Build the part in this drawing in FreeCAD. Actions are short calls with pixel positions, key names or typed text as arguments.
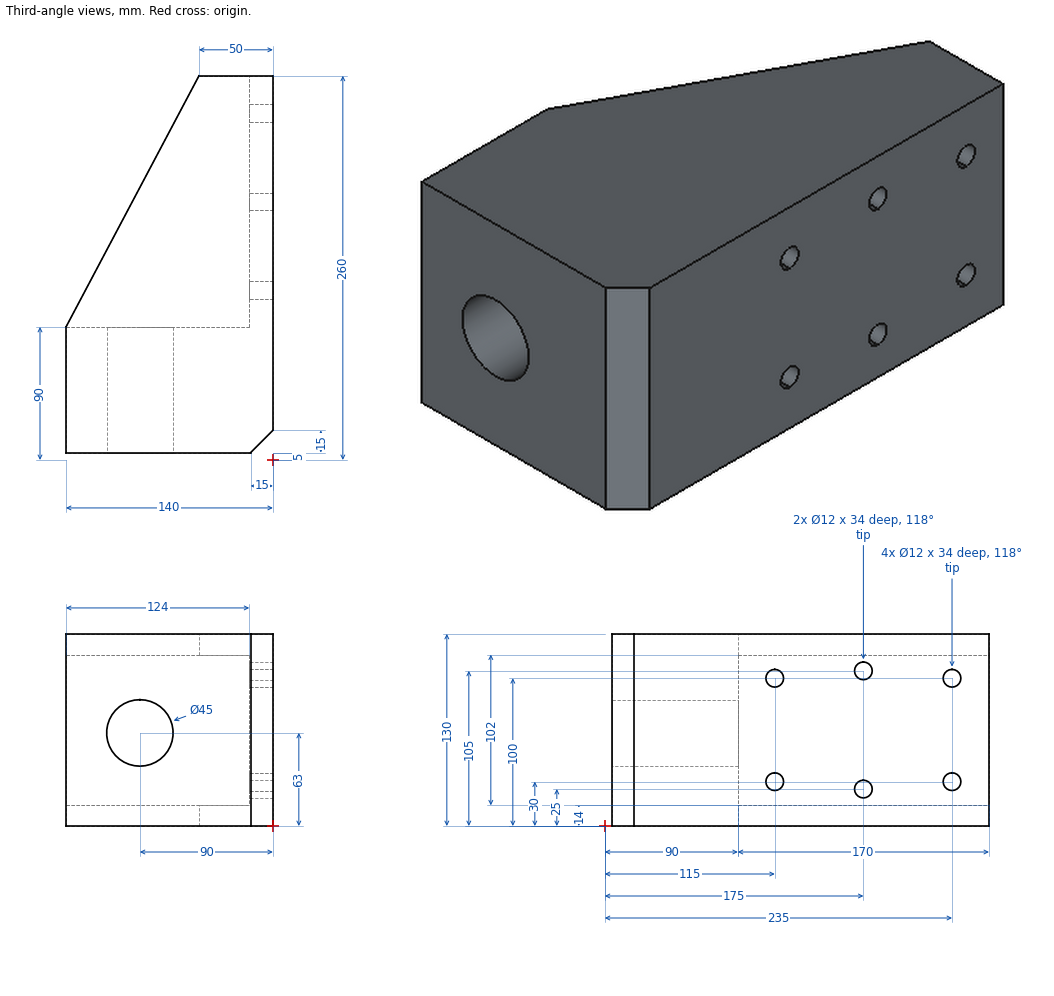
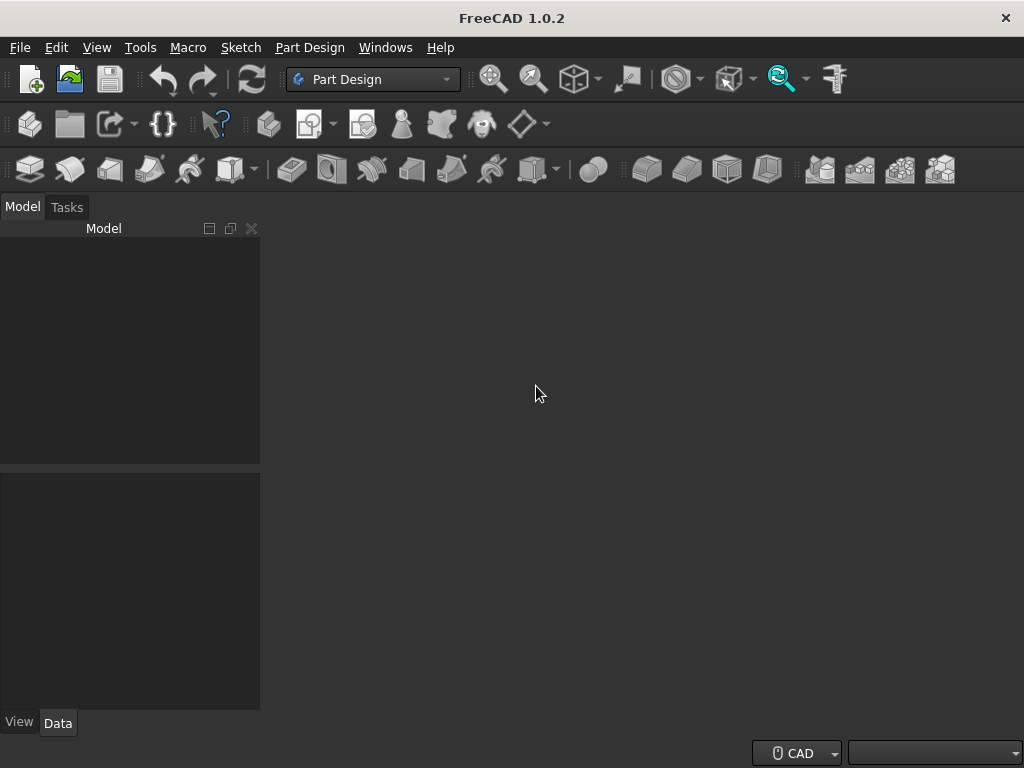
click(30, 80)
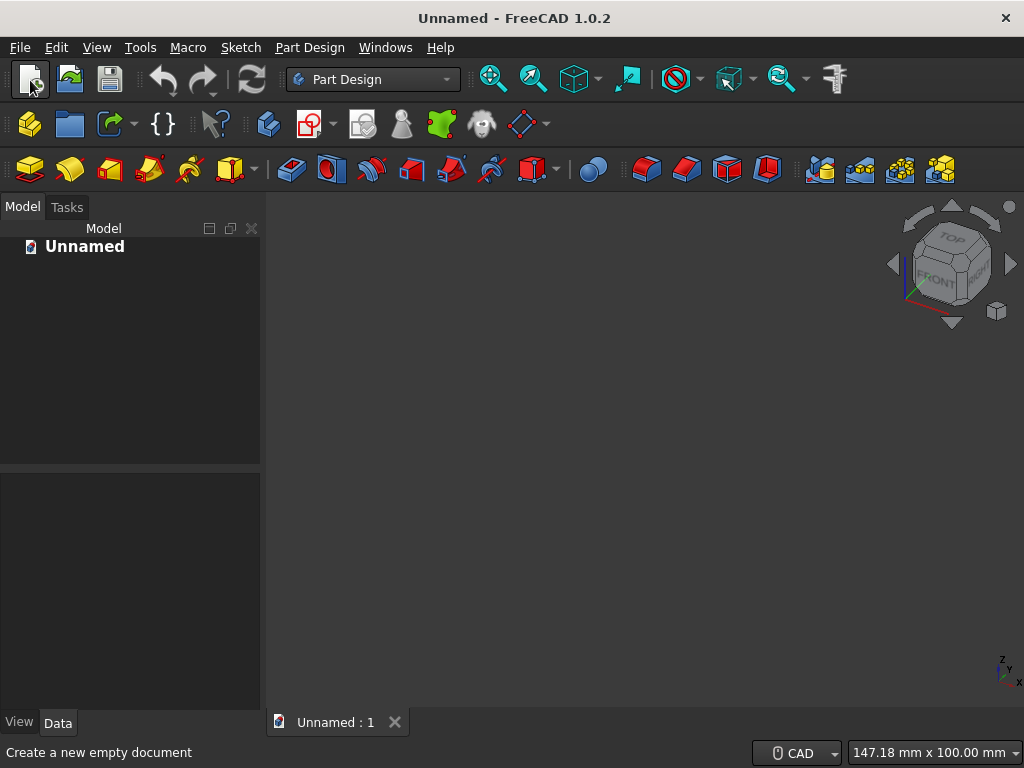
click(310, 124)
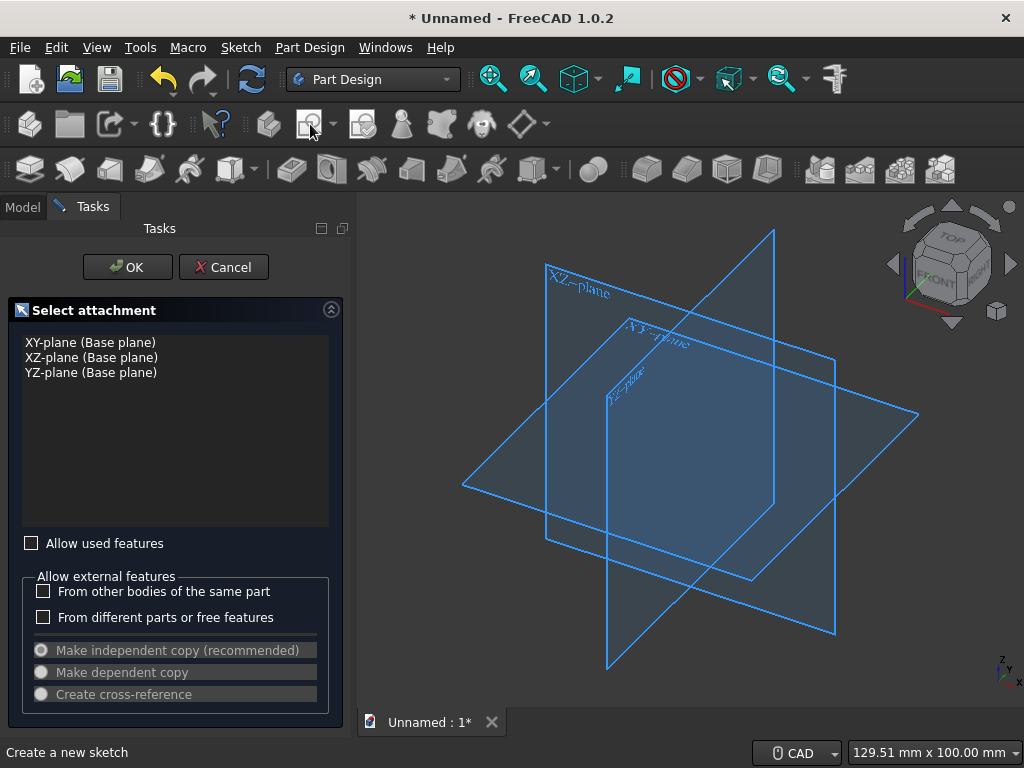
click(82, 342)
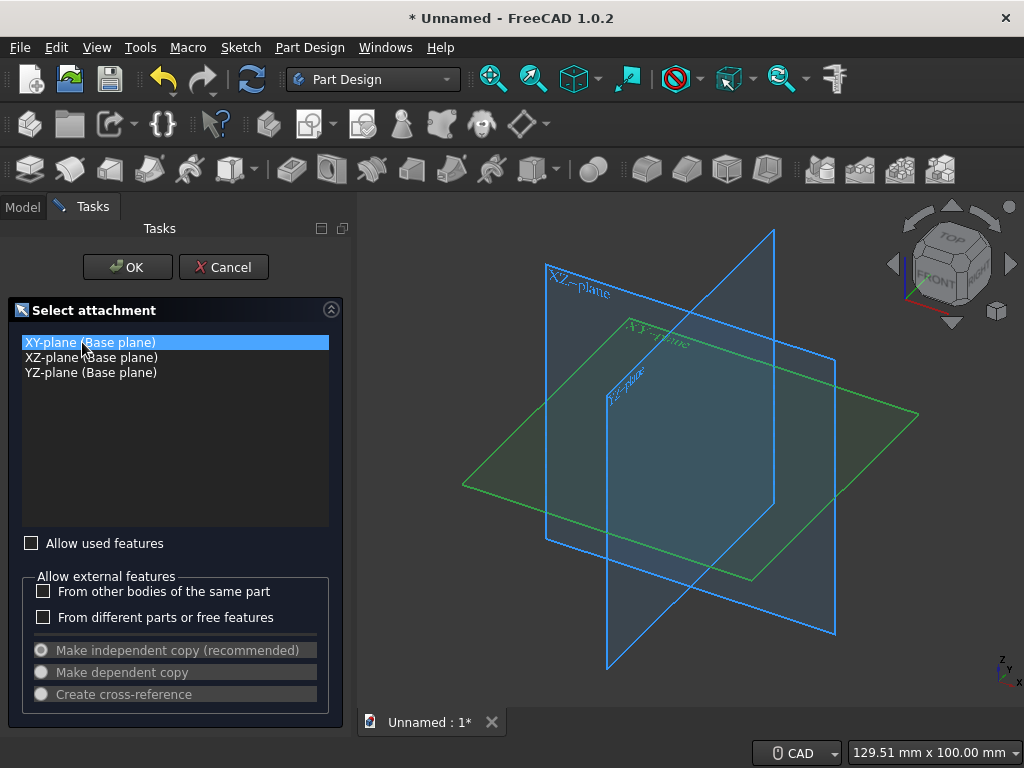
click(128, 267)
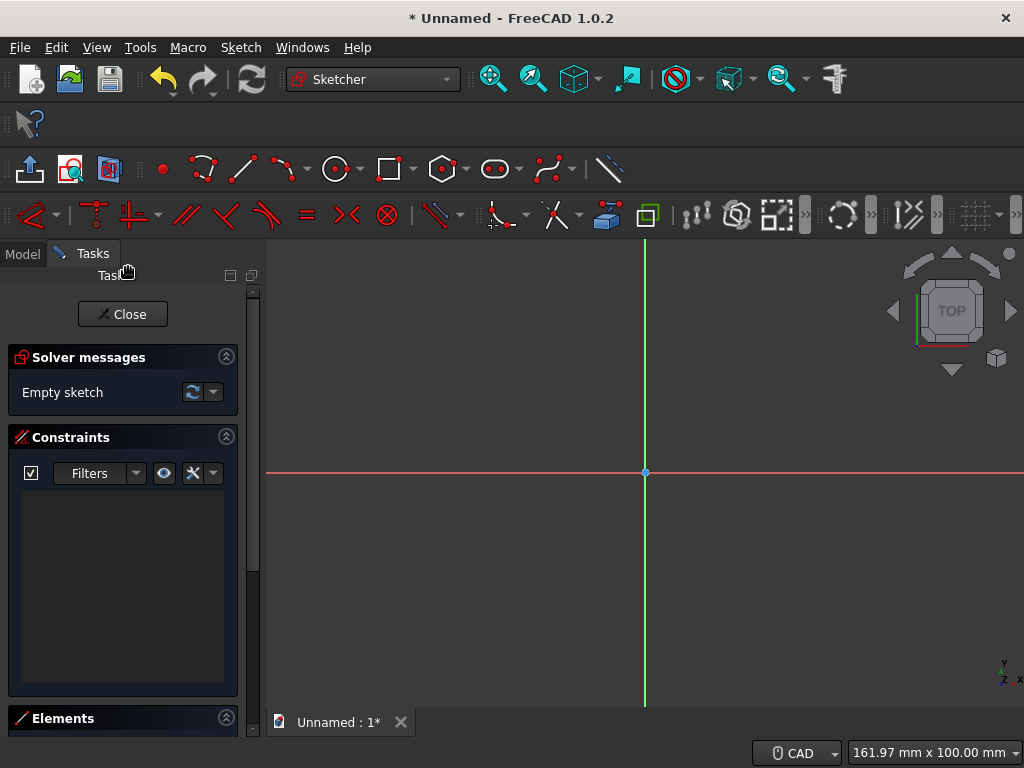
scroll(661, 672, down, 7)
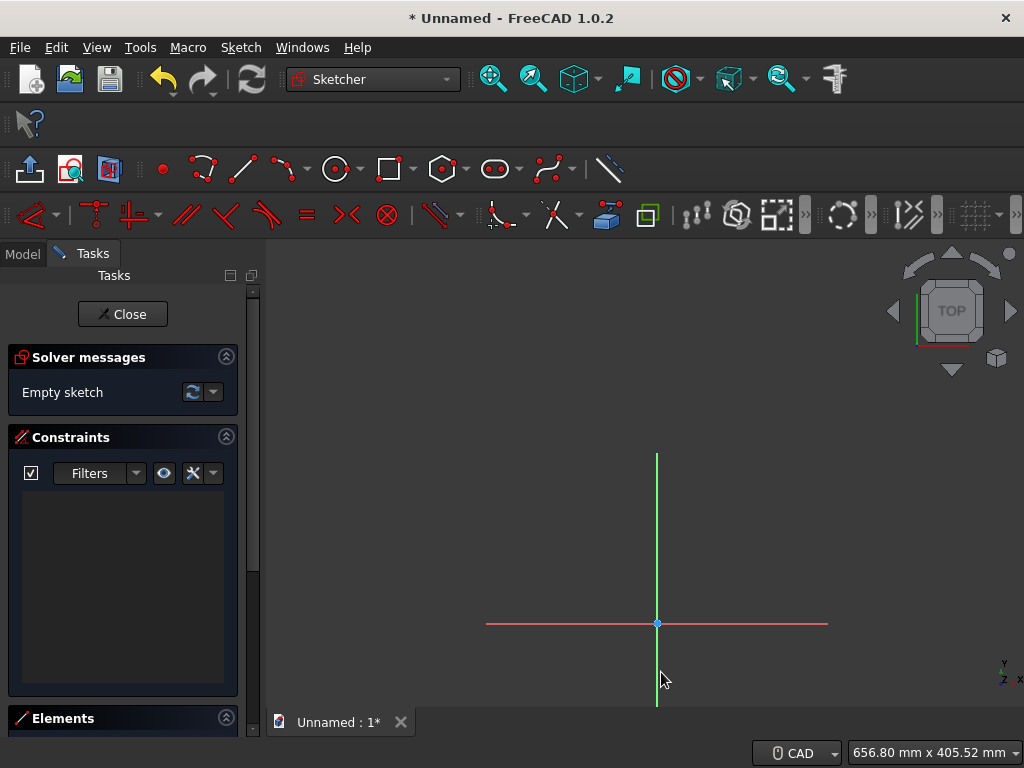
click(204, 170)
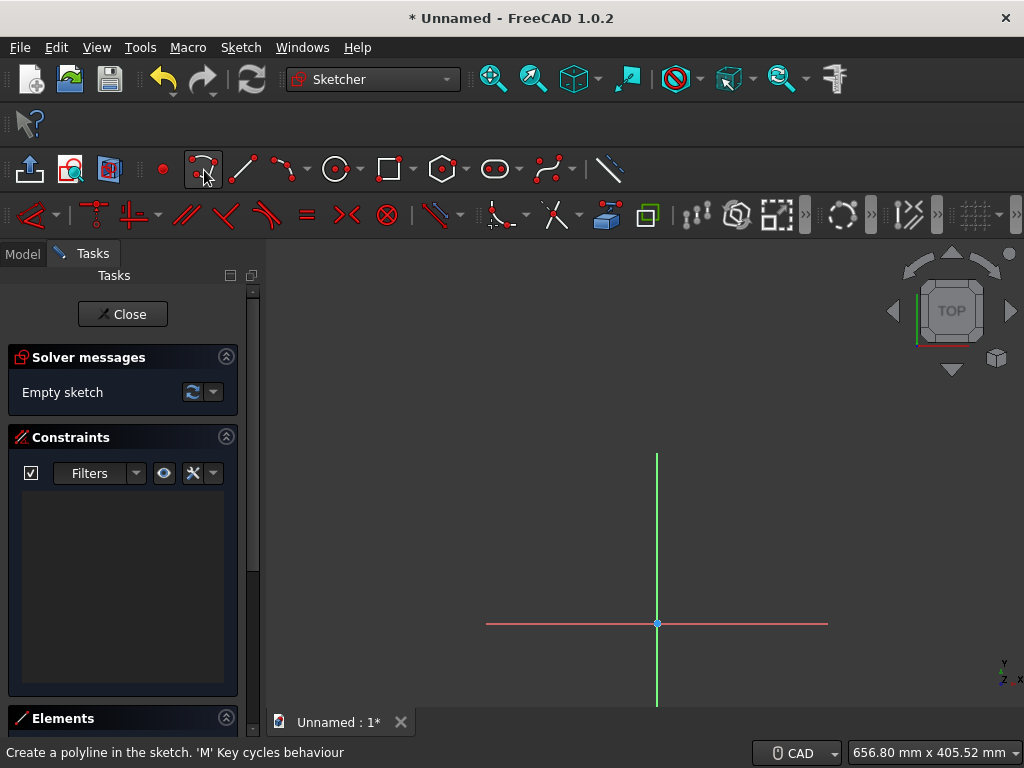
click(657, 624)
click(648, 324)
click(600, 324)
click(496, 520)
click(496, 615)
click(657, 624)
key(Escape)
key(Escape)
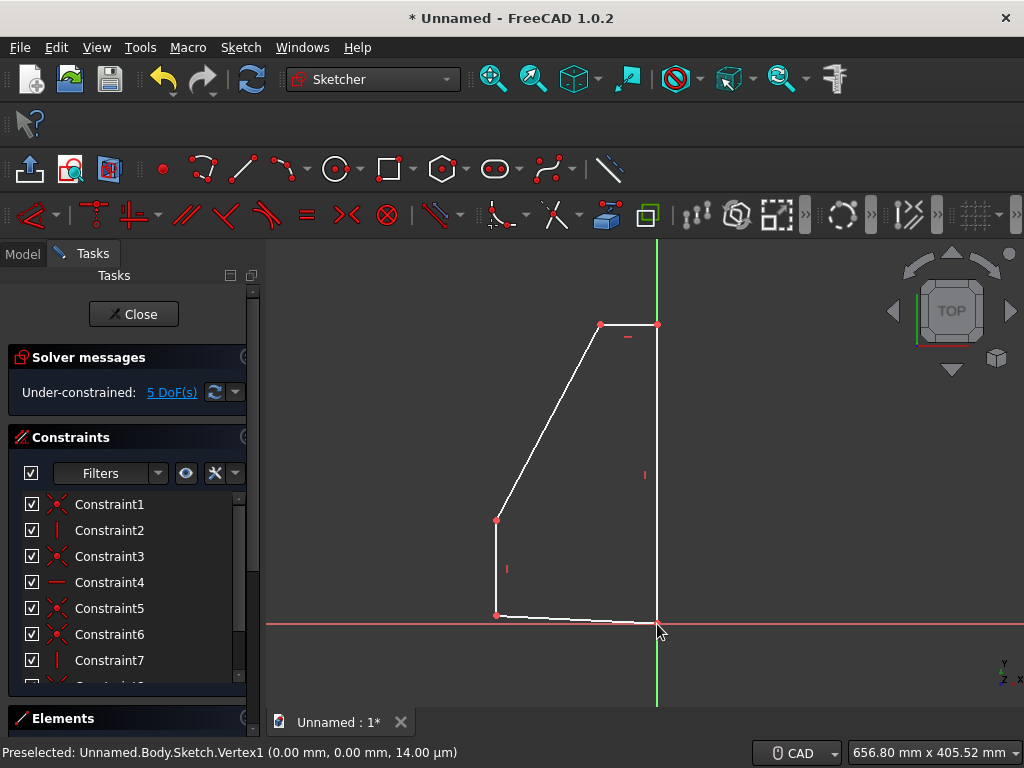
click(609, 621)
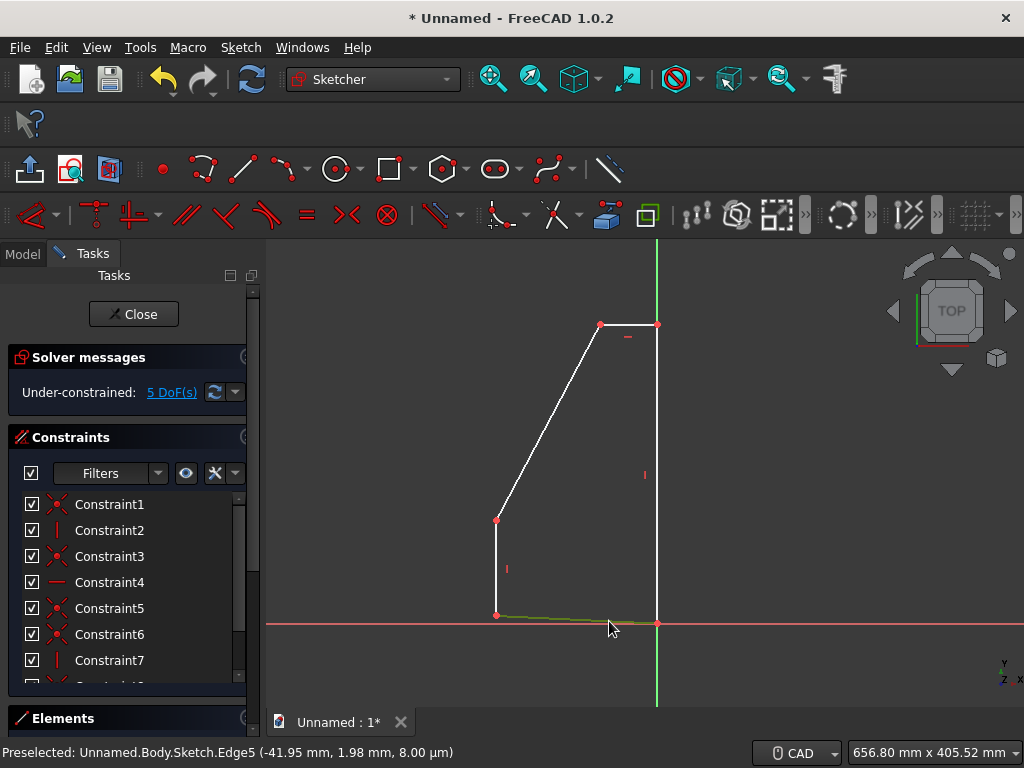
key(h)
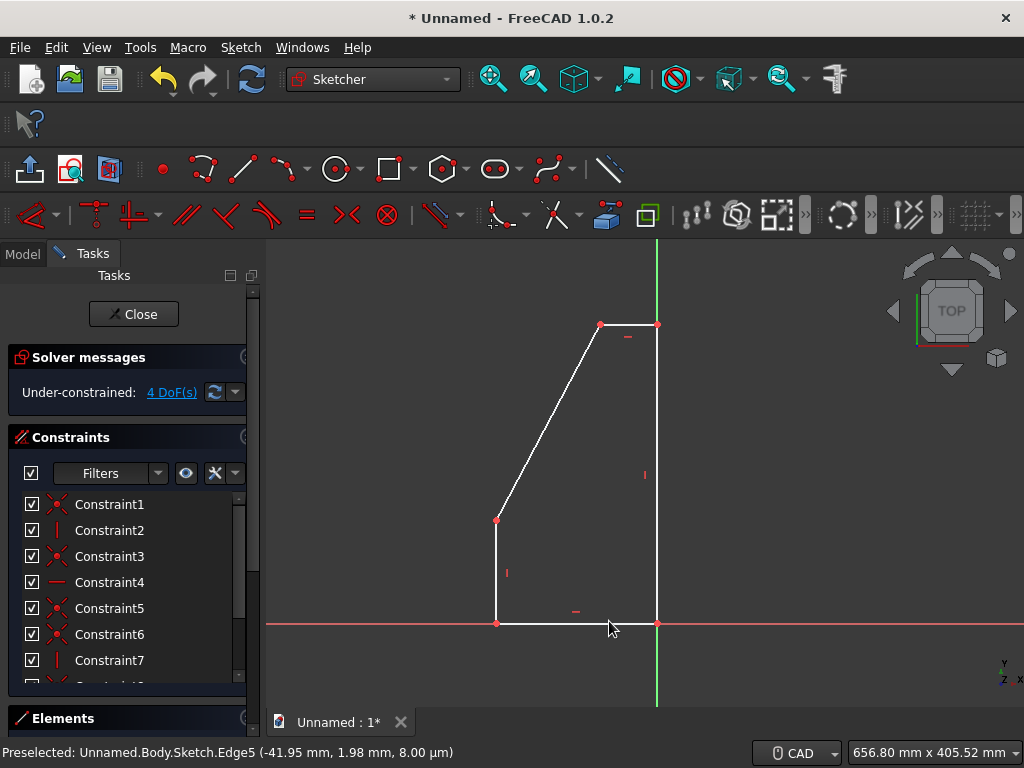
click(32, 216)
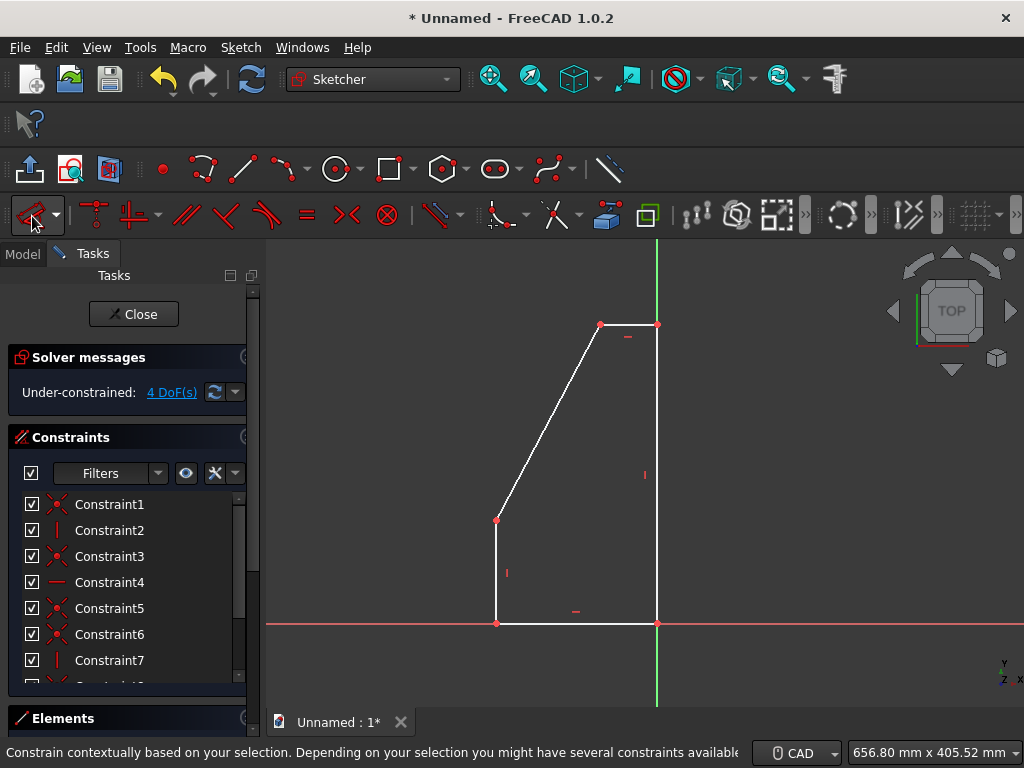
click(640, 325)
click(629, 291)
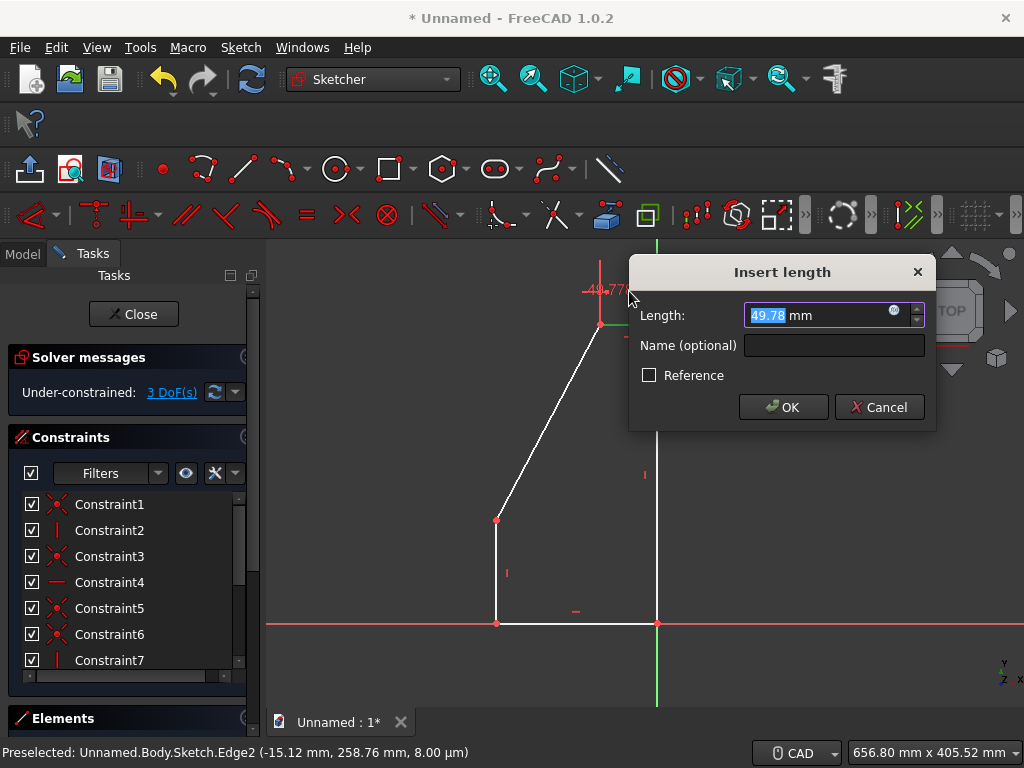
text(50)
key(Return)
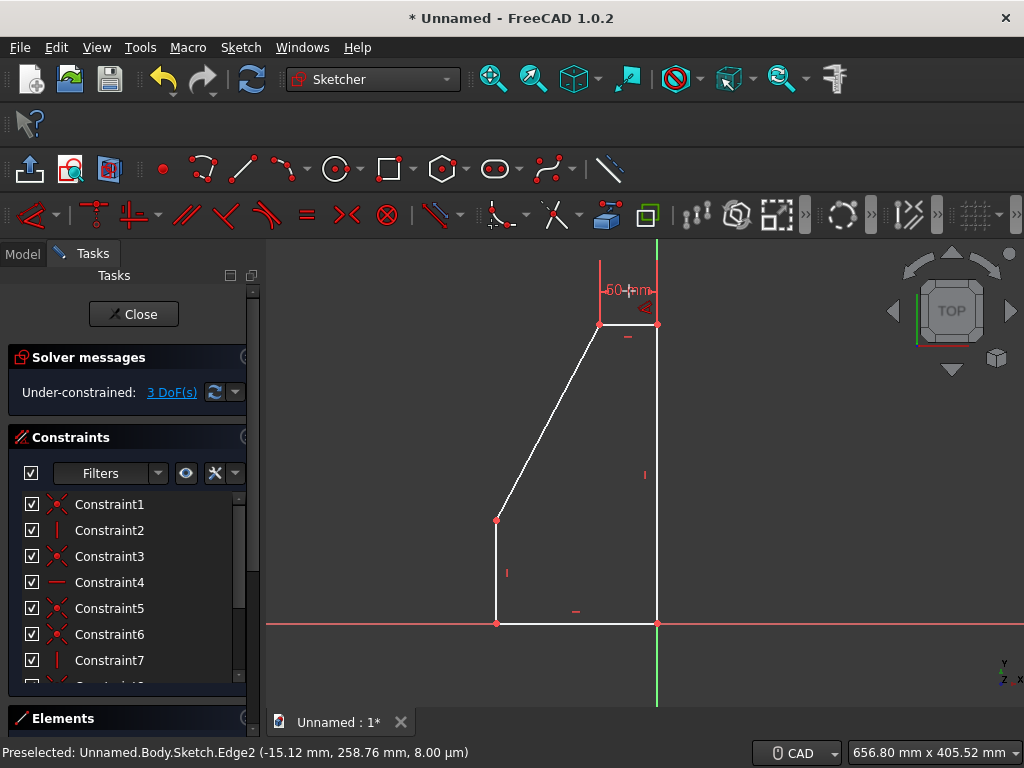
click(496, 552)
click(462, 572)